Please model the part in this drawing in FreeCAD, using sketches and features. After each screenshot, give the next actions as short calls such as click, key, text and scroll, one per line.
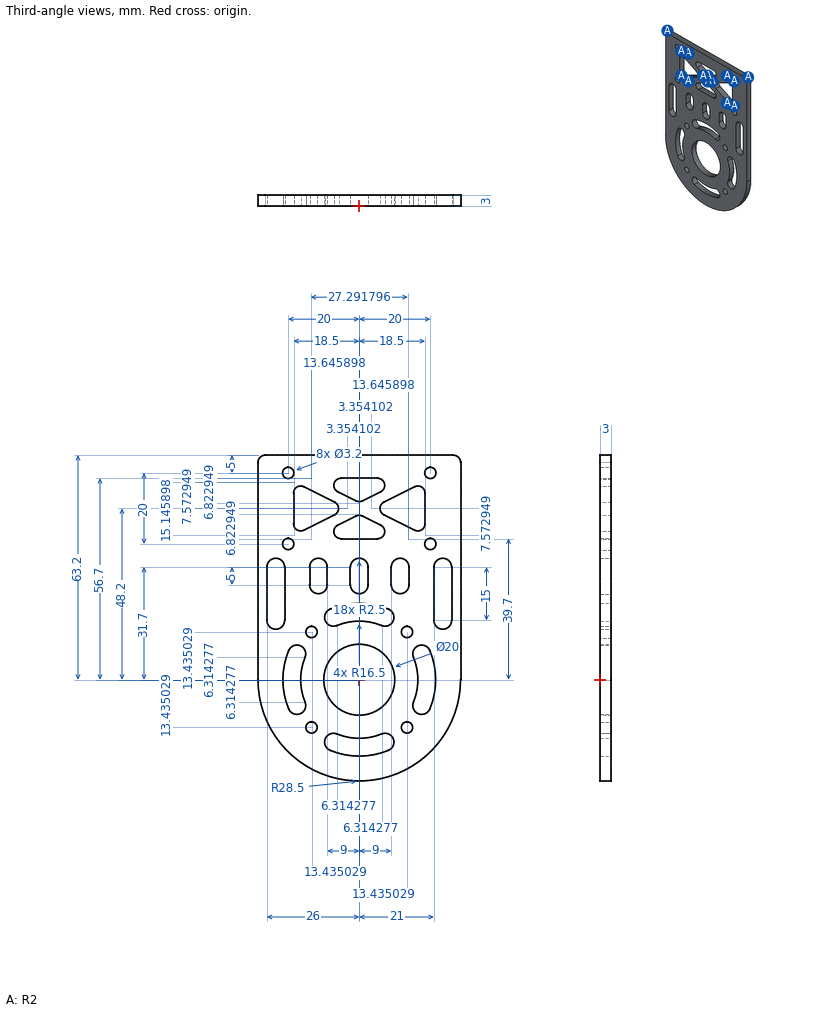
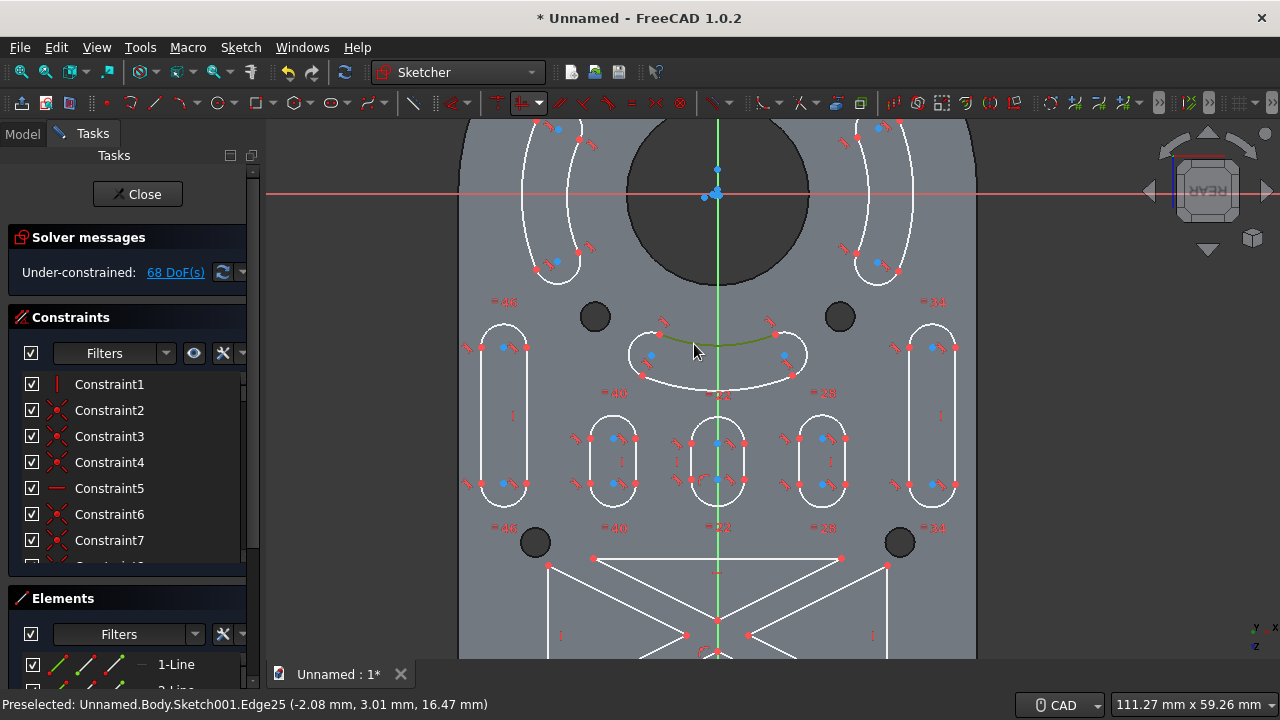
click(569, 172)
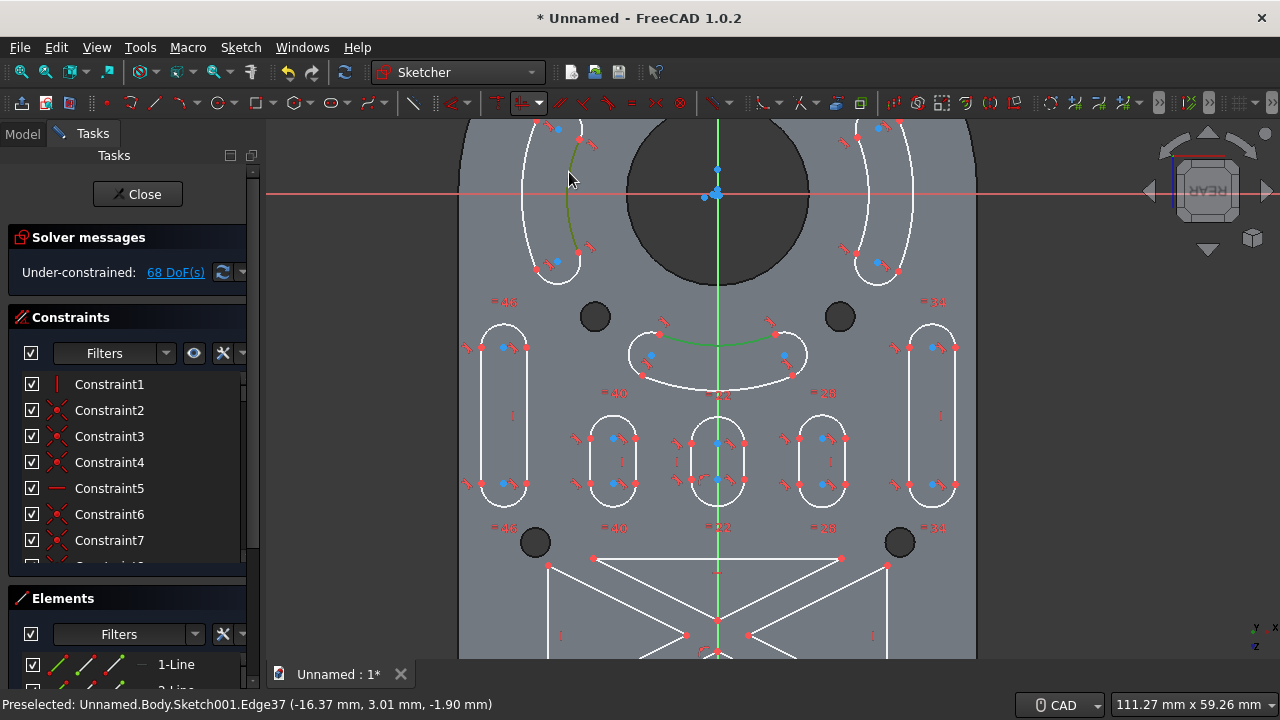
key(c)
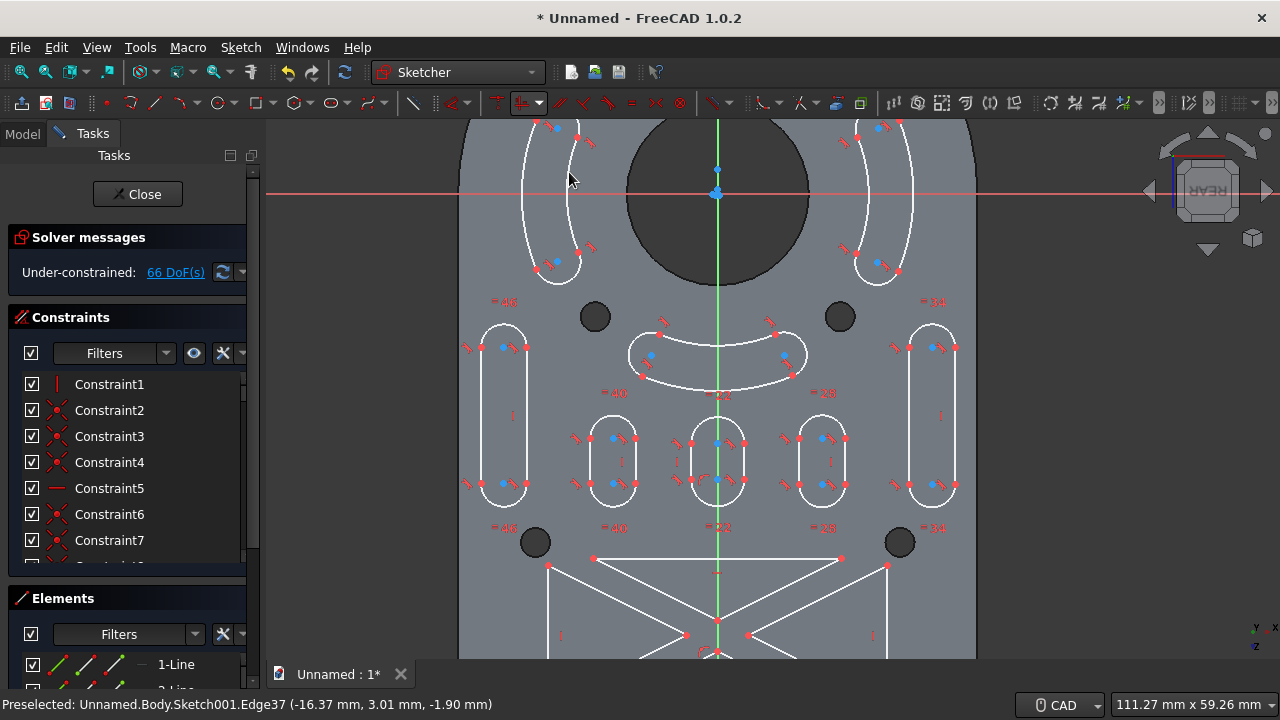
click(694, 344)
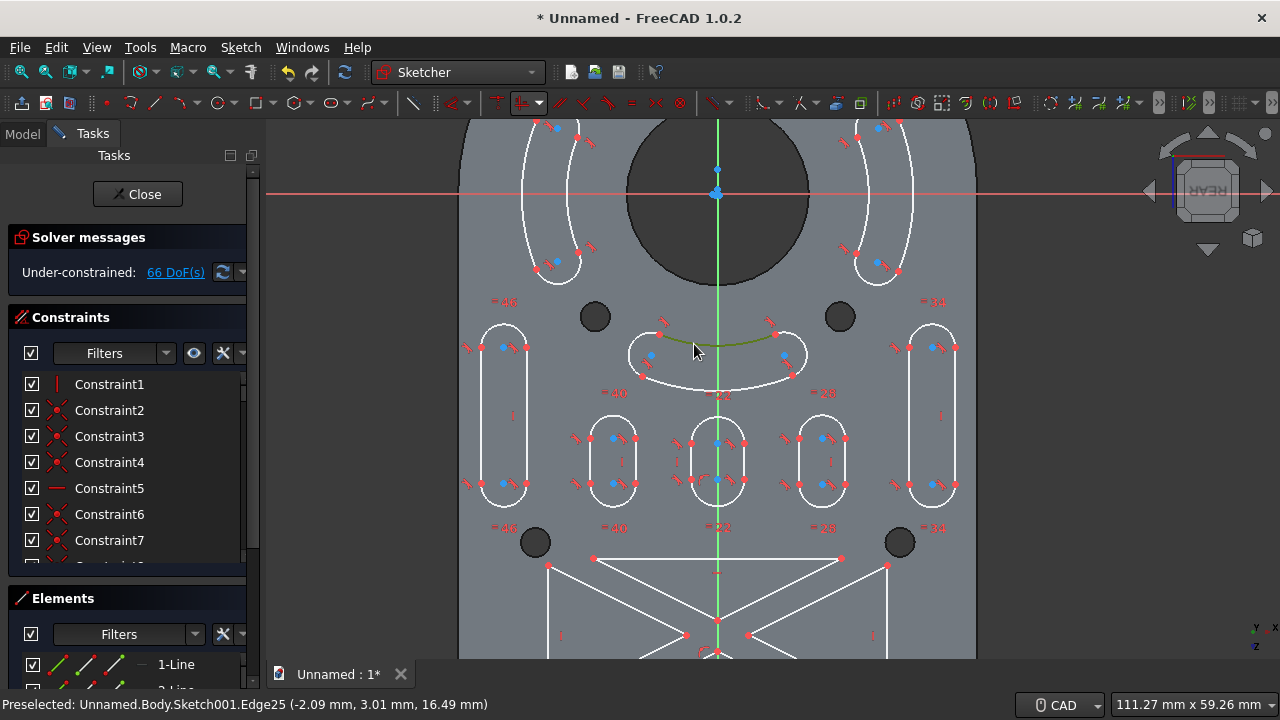
click(524, 165)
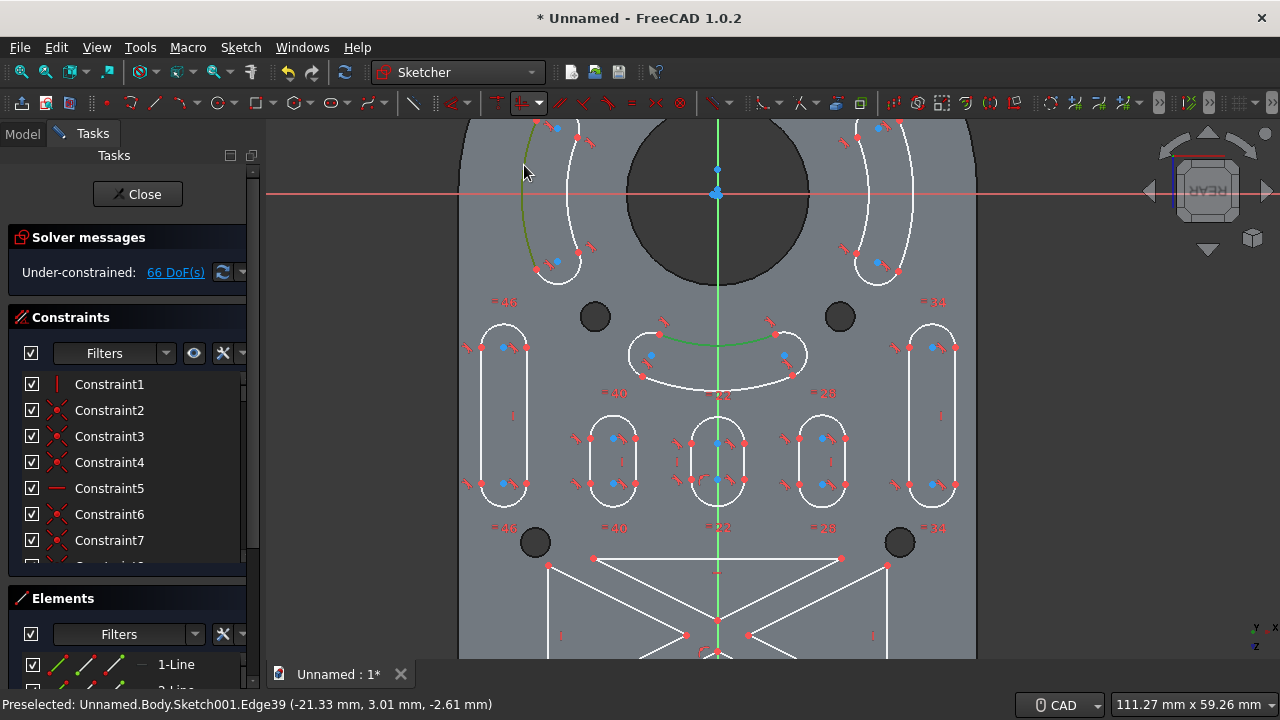
key(c)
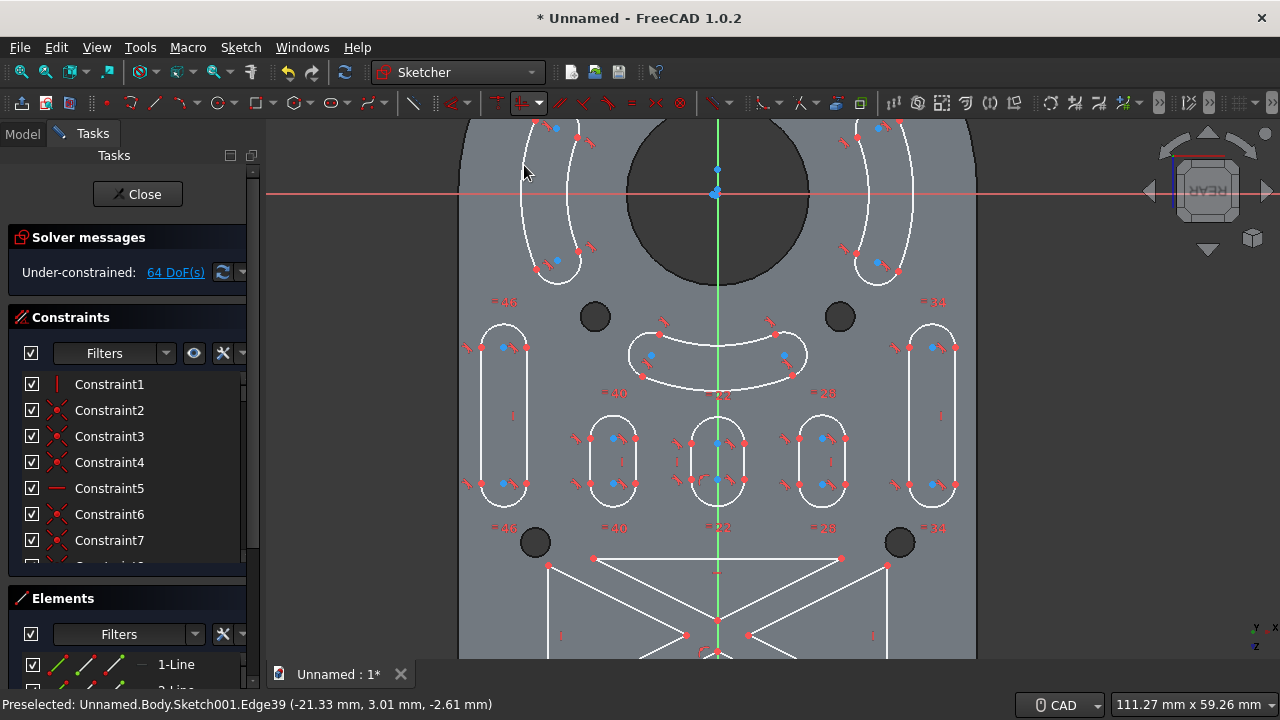
click(694, 344)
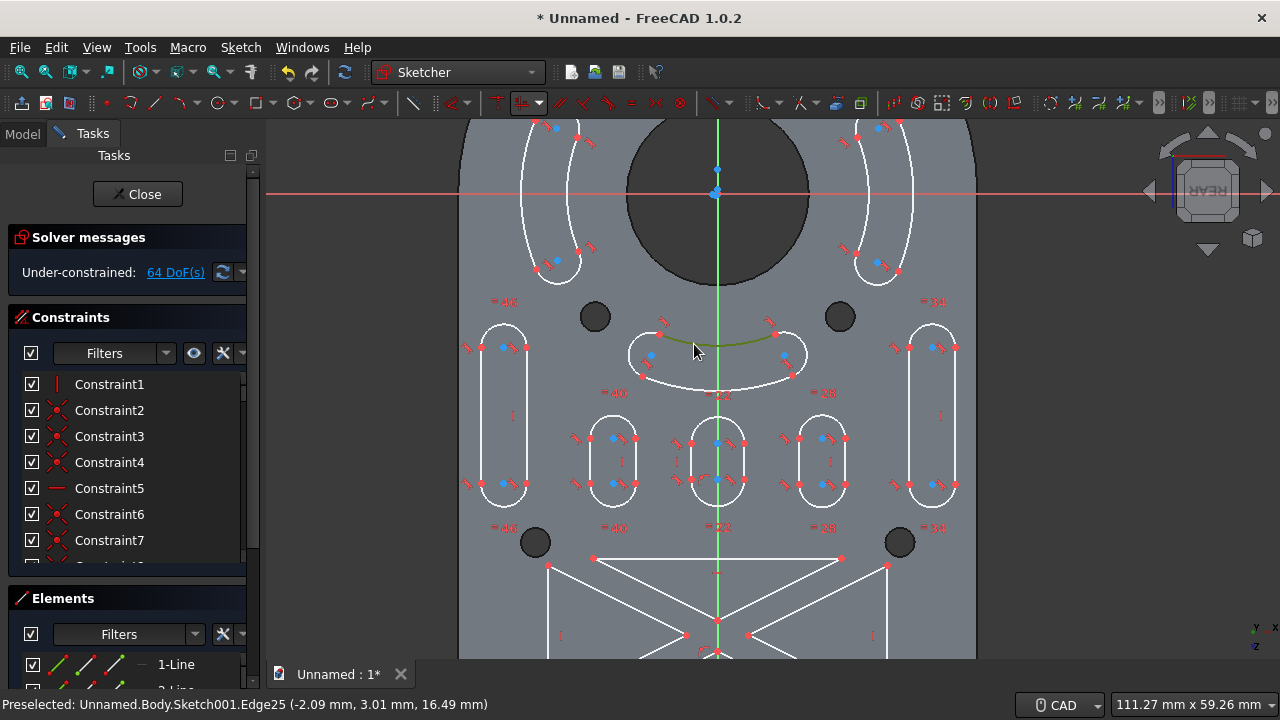
click(867, 219)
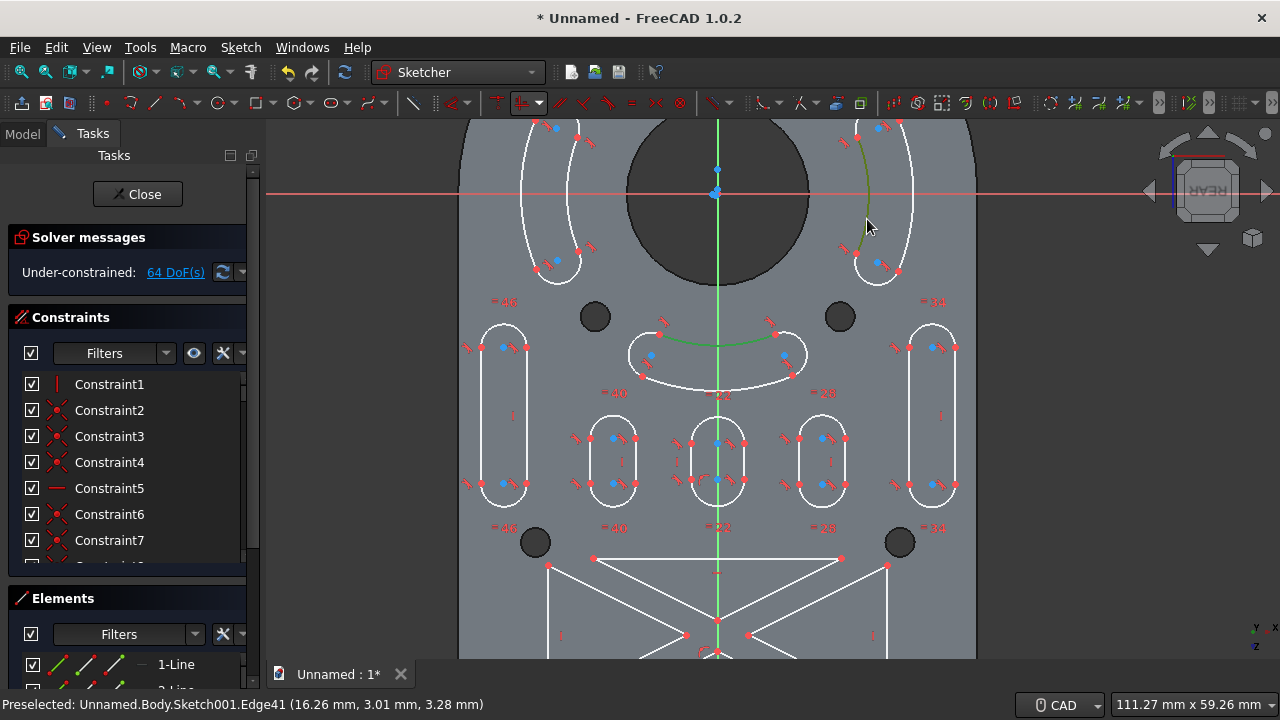
key(c)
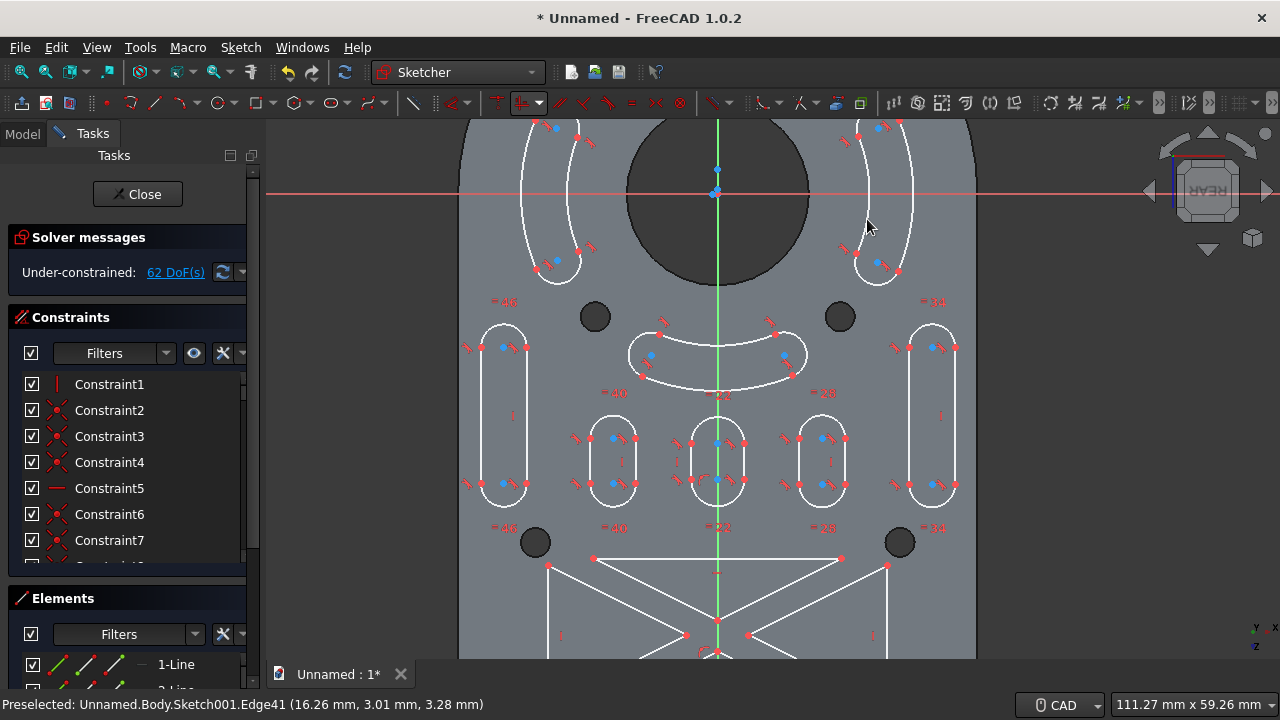
click(694, 344)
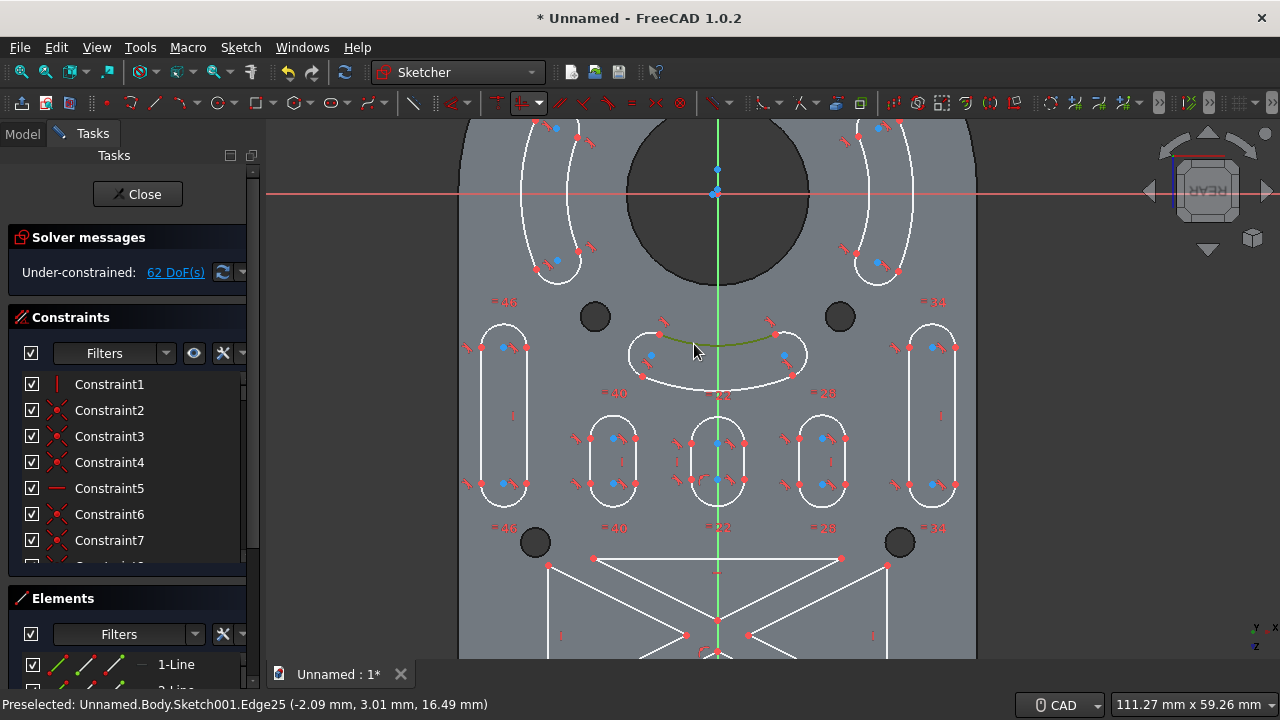
click(911, 227)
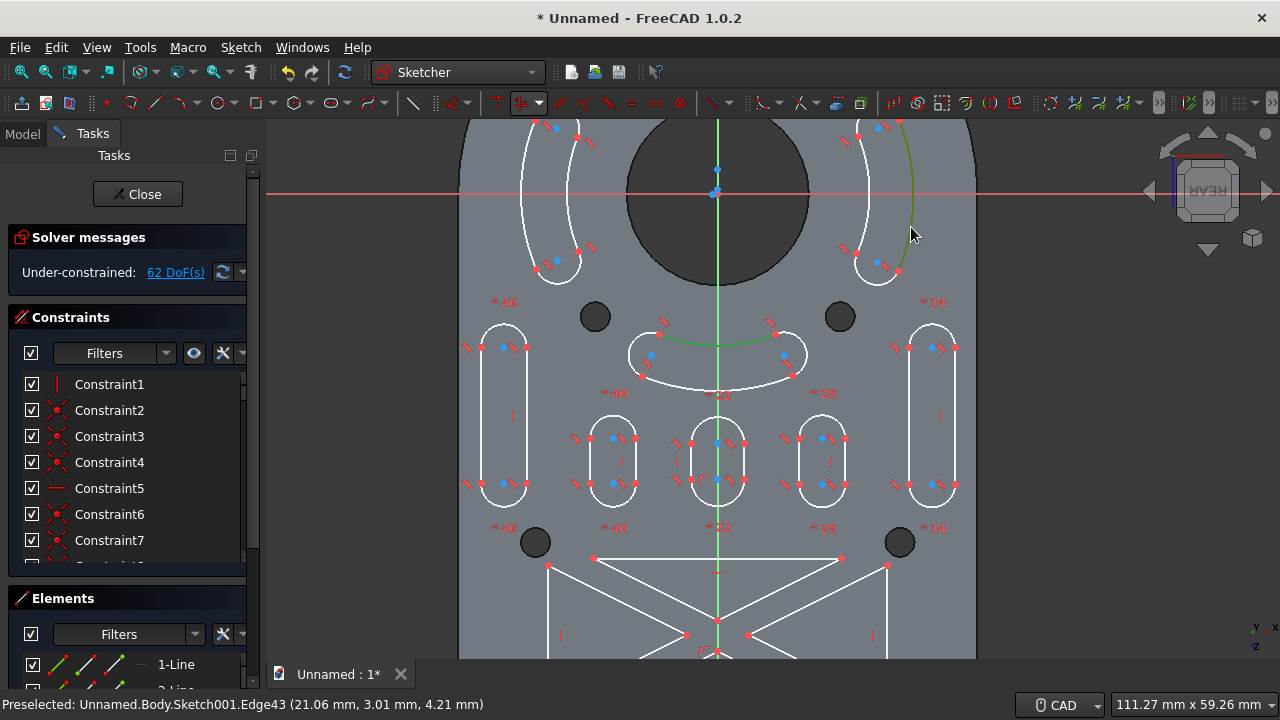
click(498, 104)